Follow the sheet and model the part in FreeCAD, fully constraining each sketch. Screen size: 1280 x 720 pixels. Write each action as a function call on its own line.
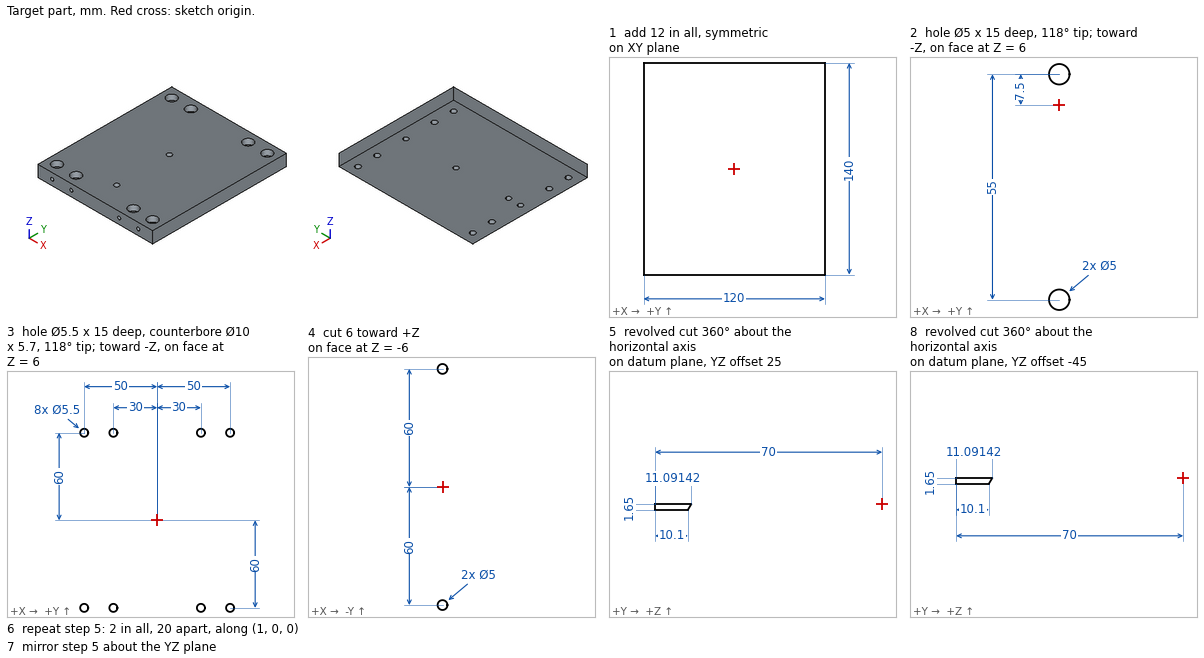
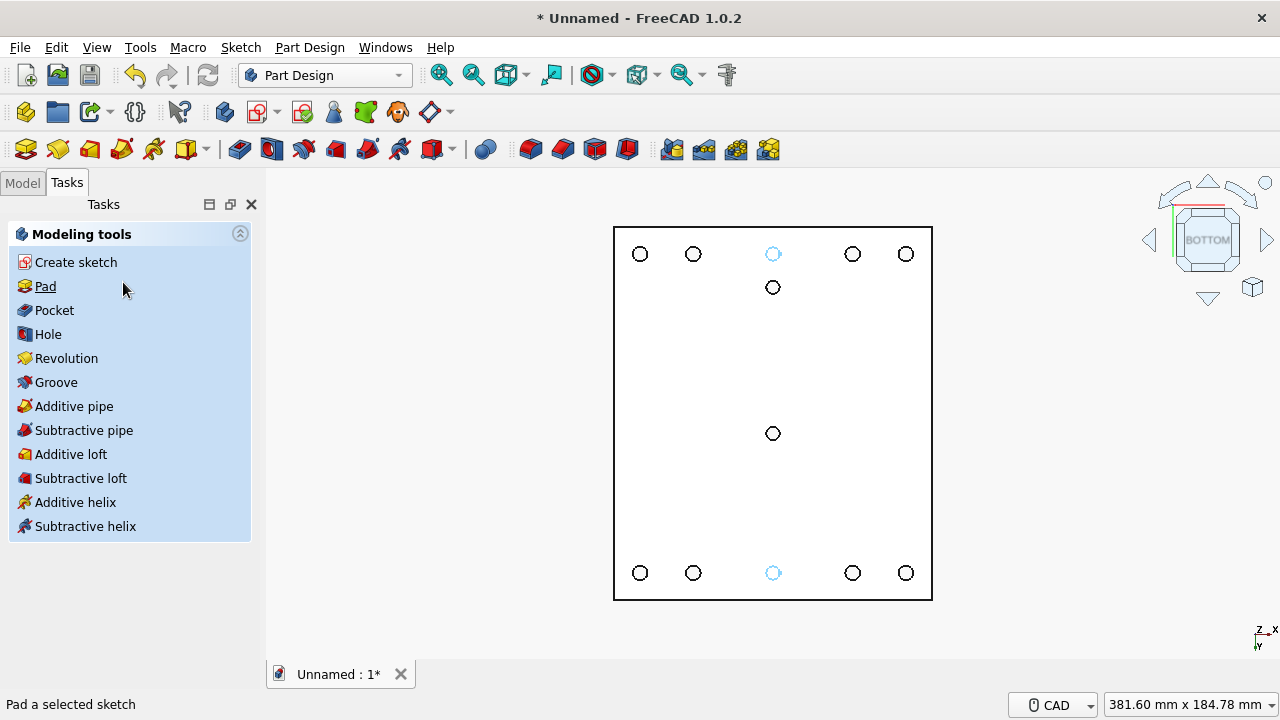
click(240, 150)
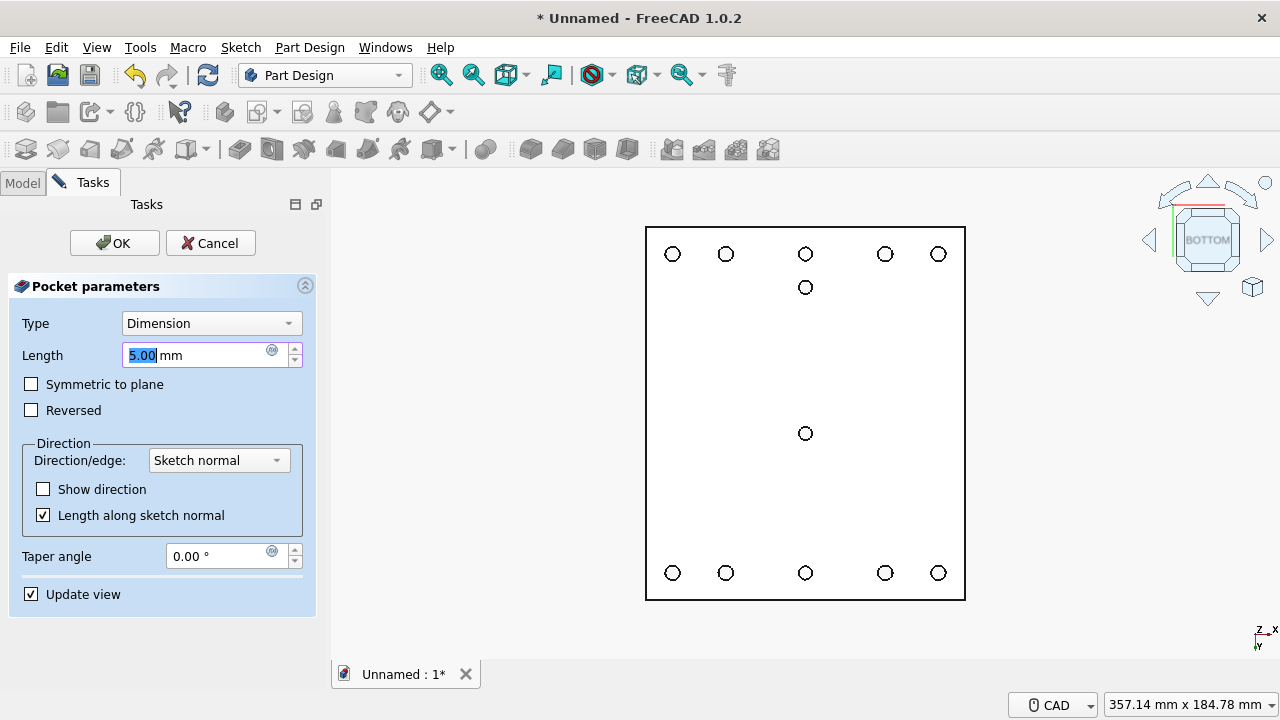
text(6)
key(Tab)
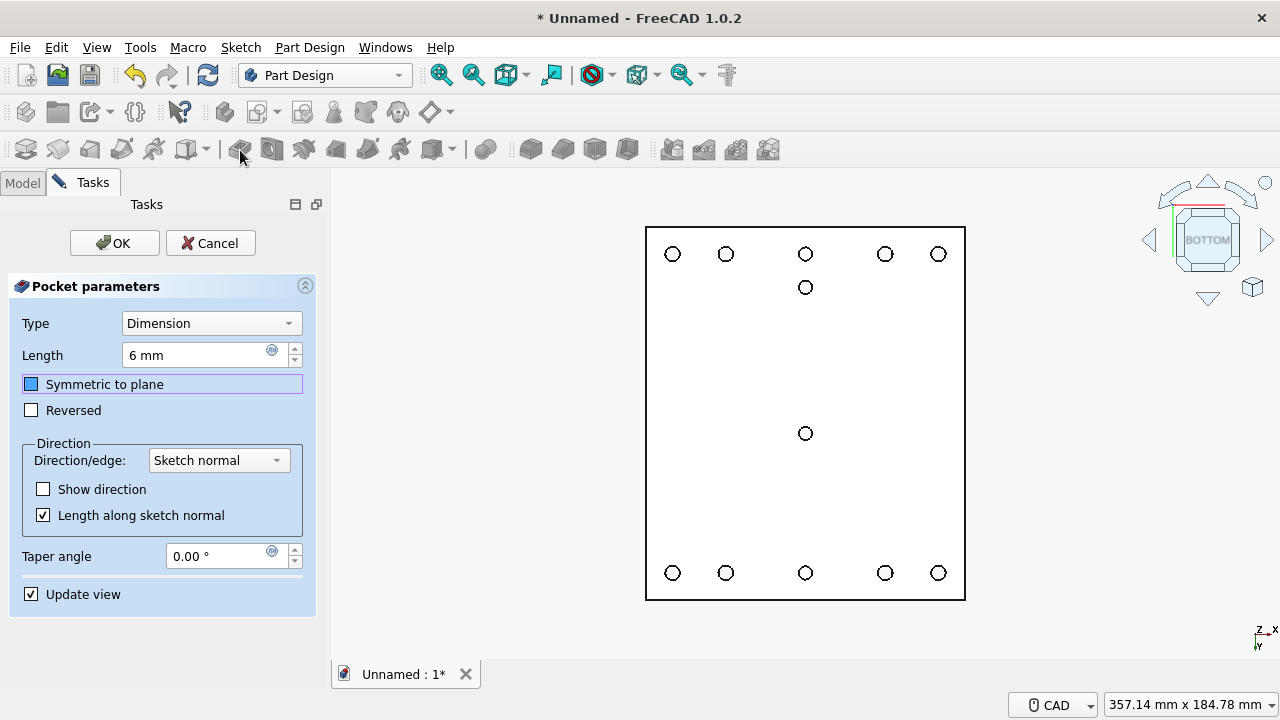
click(115, 243)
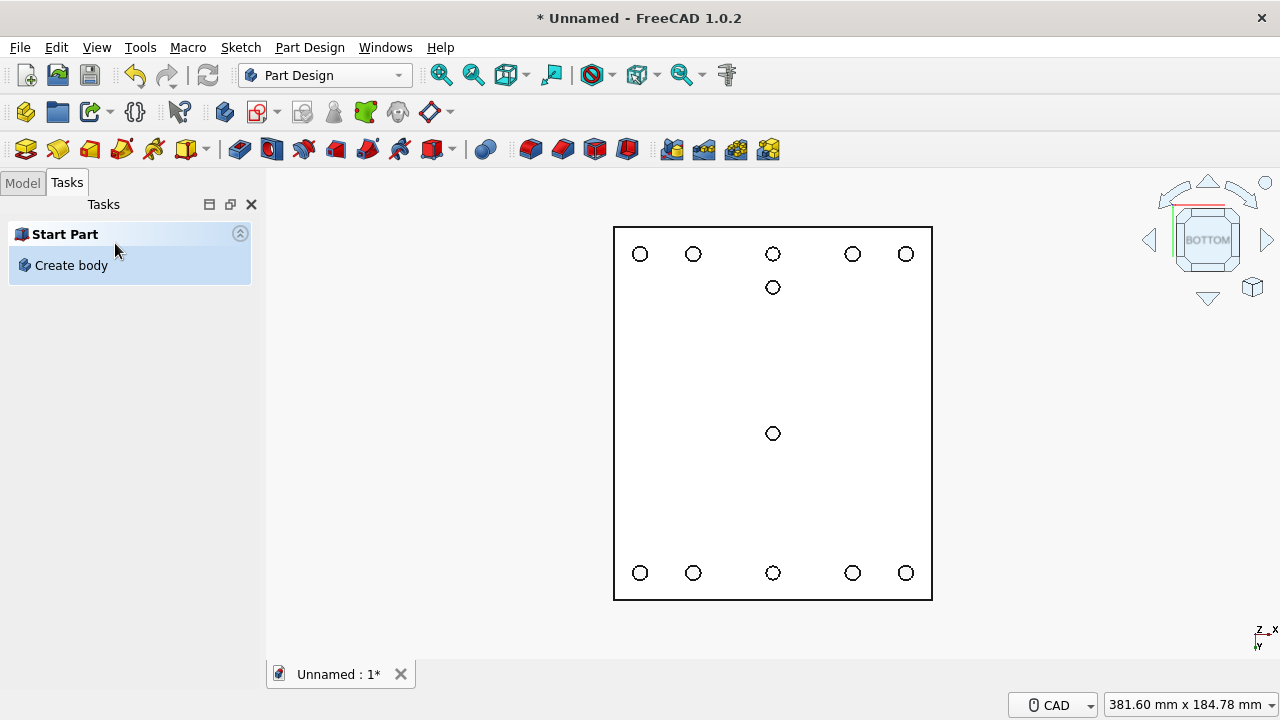
click(23, 182)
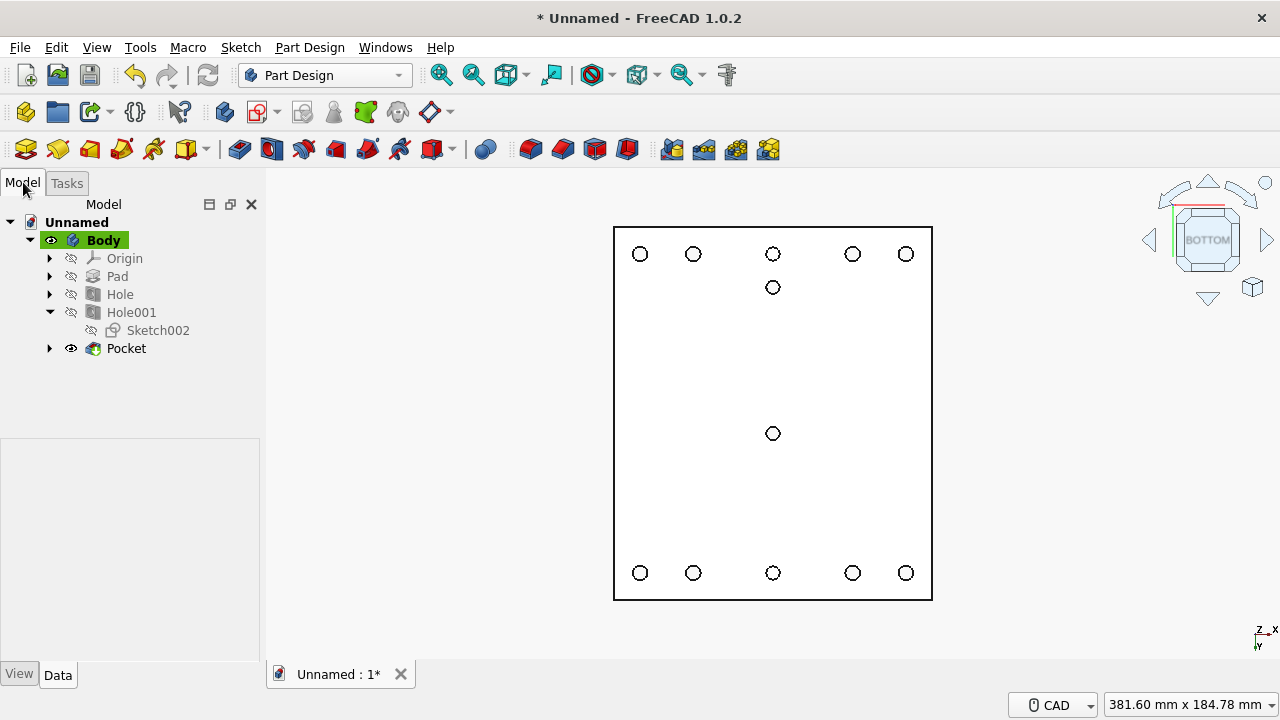
click(50, 258)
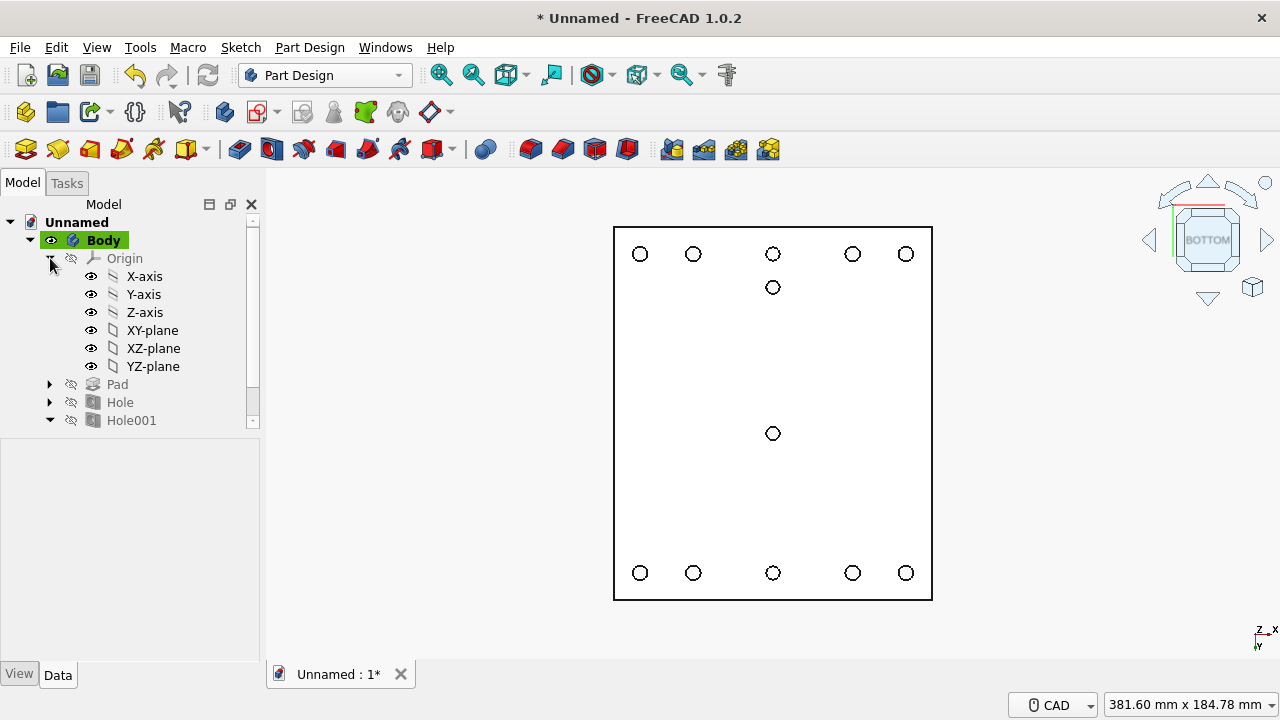
click(136, 366)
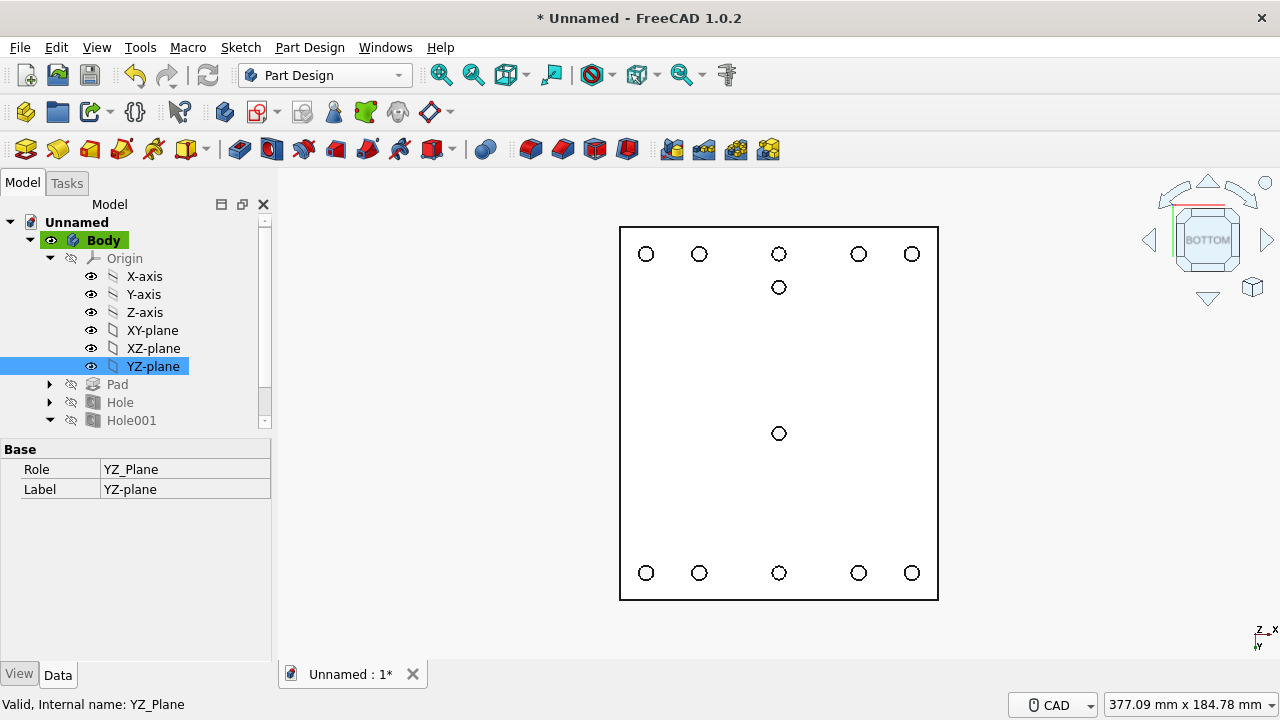
click(430, 112)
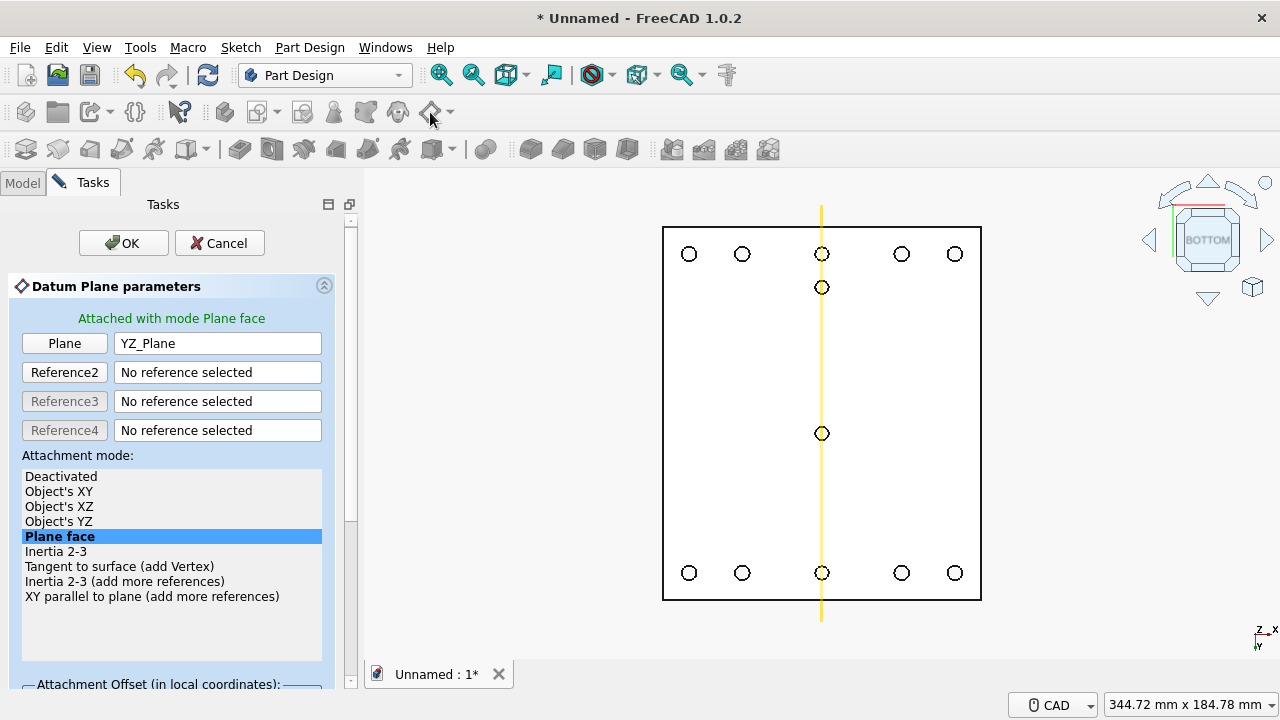
scroll(351, 451, down, 3)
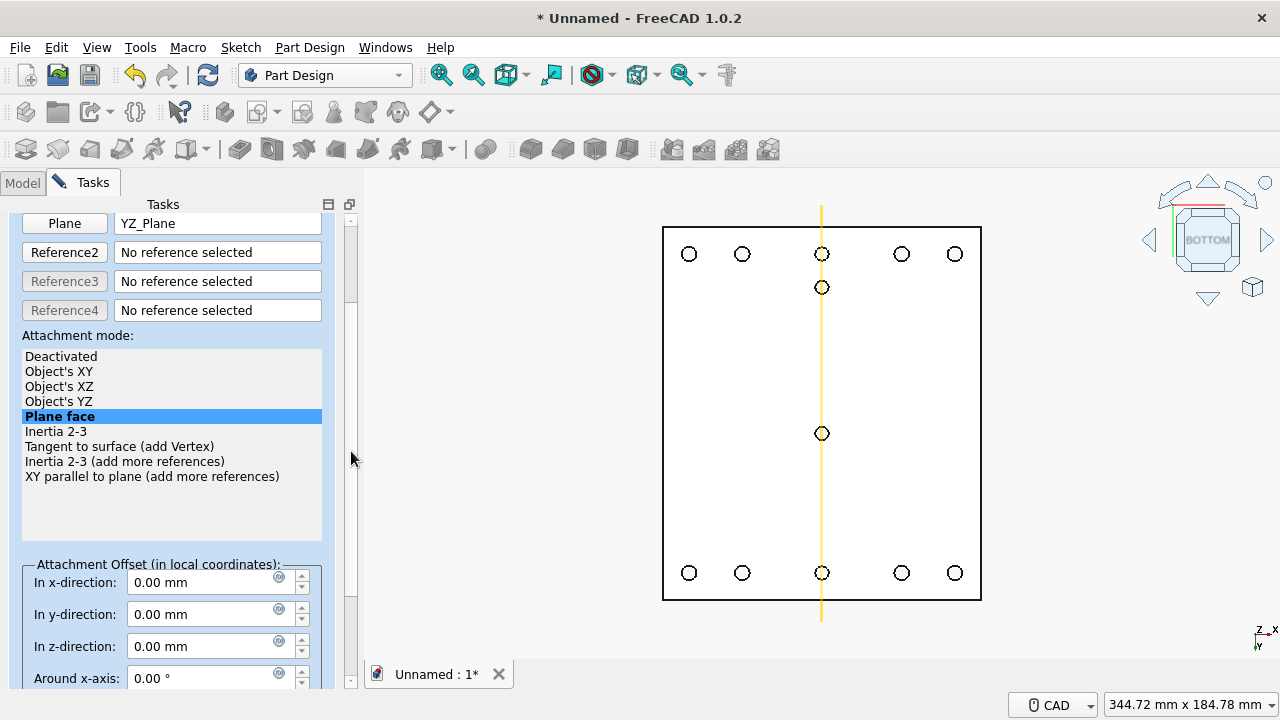
triple_click(210, 586)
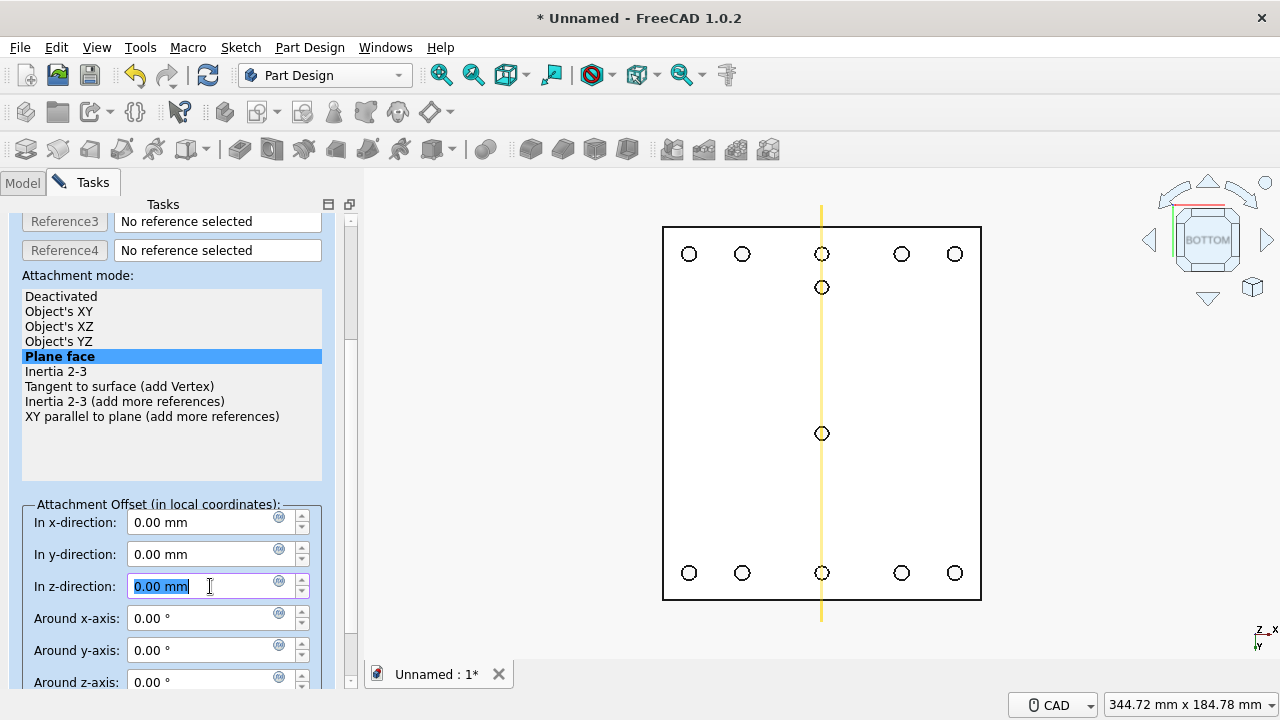
text(25)
key(Tab)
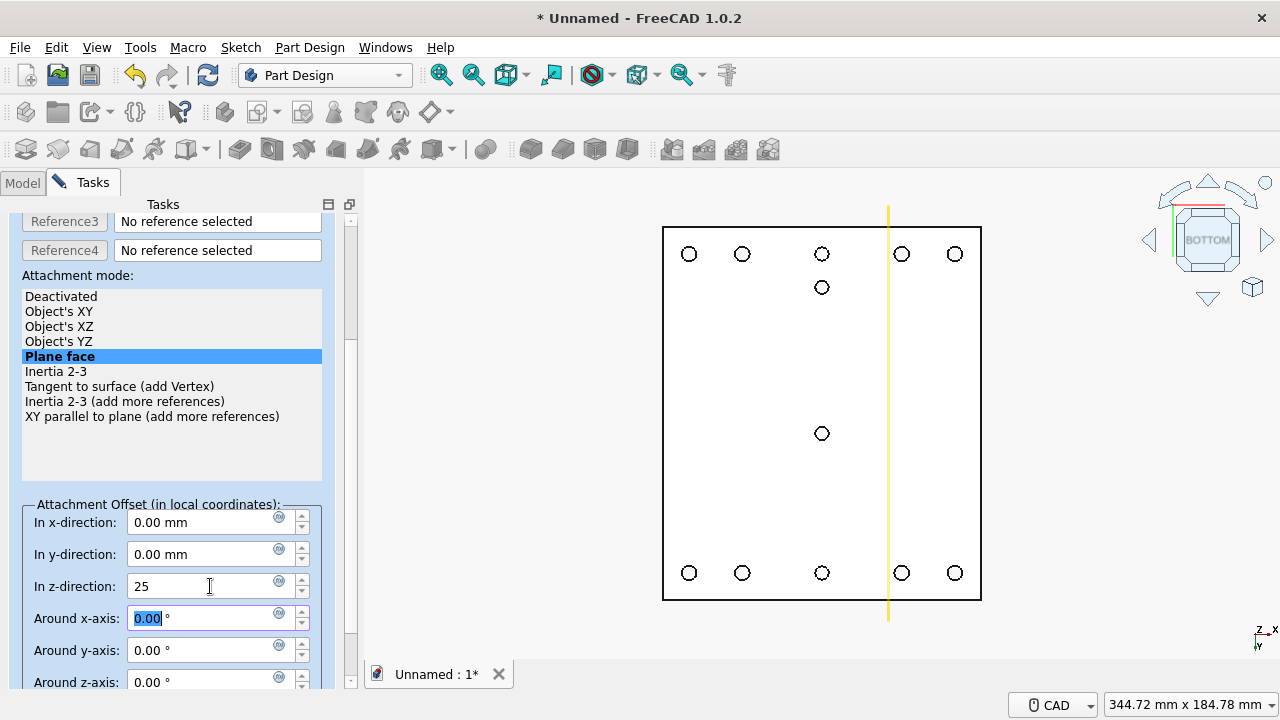
scroll(351, 451, up, 4)